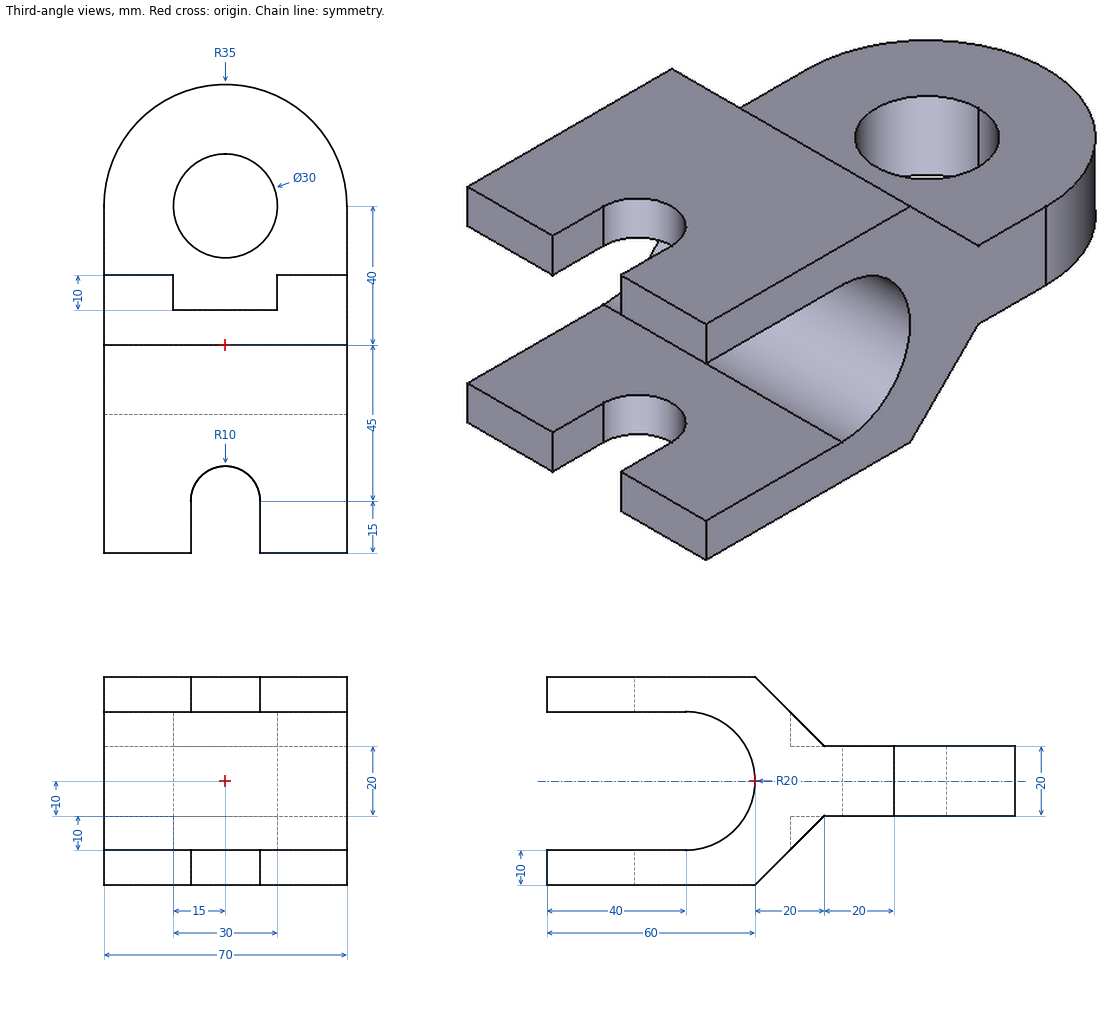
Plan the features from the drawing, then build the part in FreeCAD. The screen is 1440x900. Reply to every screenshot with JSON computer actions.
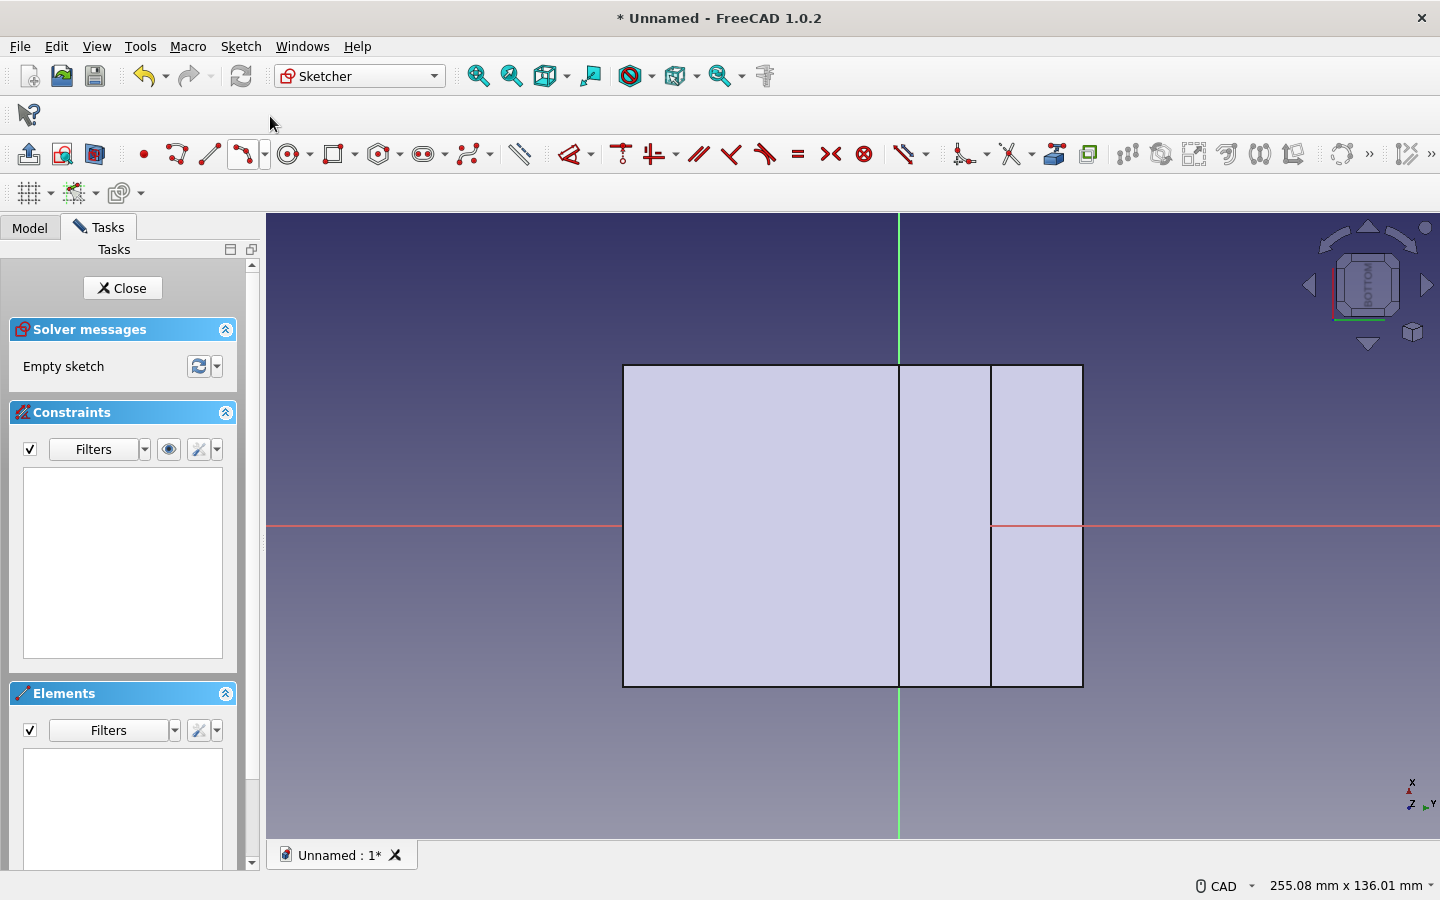
{"action": "key", "text": "g l"}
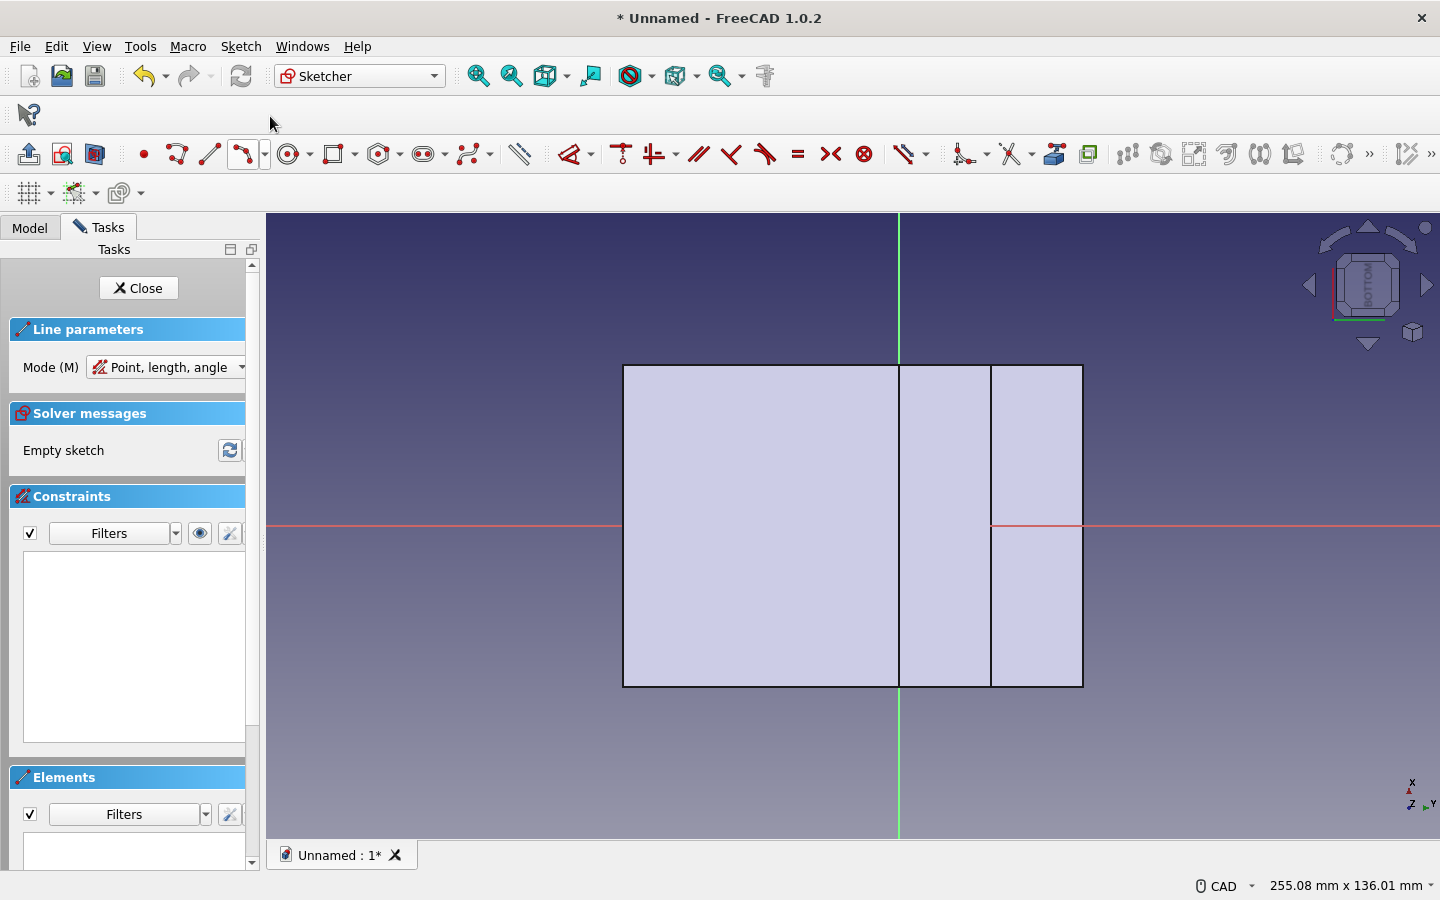
{"action": "left_click", "coordinate": [1083, 365]}
{"action": "left_click", "coordinate": [1083, 687]}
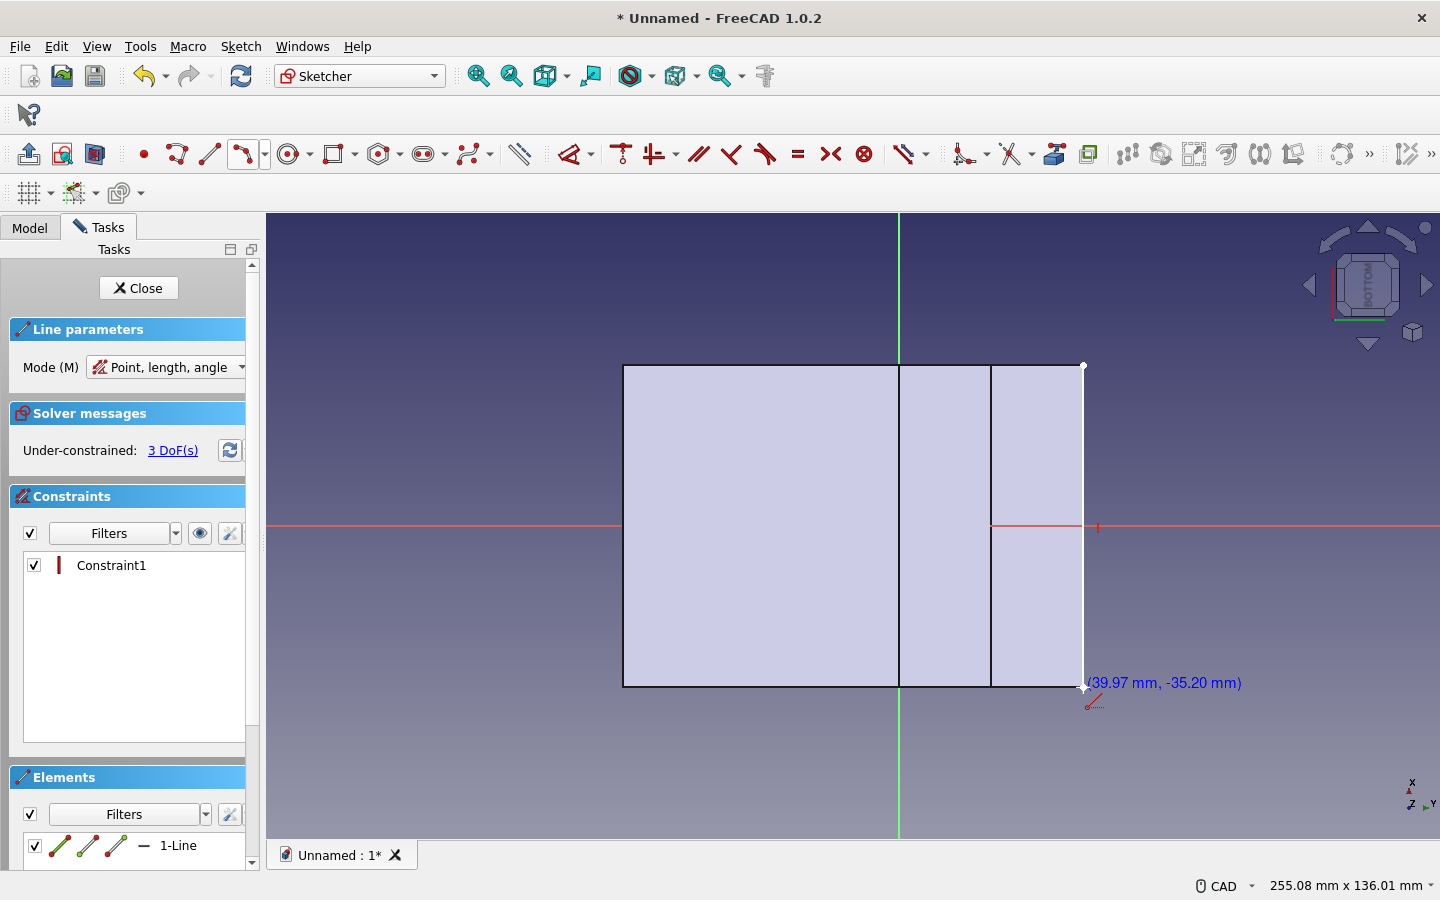
{"action": "left_click", "coordinate": [242, 154]}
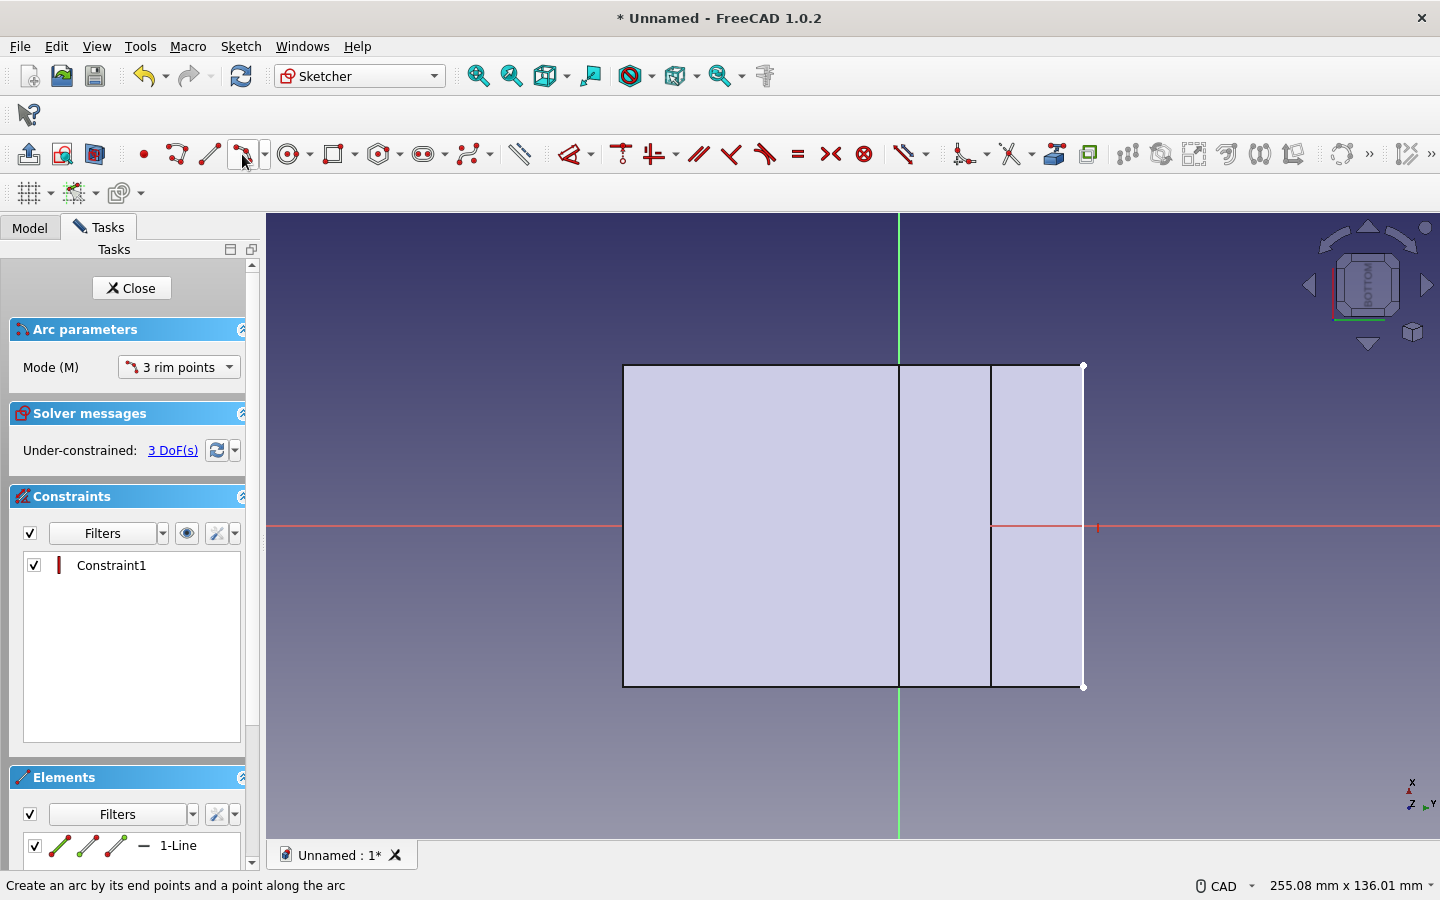
{"action": "left_click", "coordinate": [1083, 688]}
{"action": "left_click", "coordinate": [1083, 366]}
{"action": "left_click", "coordinate": [1236, 576]}
{"action": "key", "text": "Escape"}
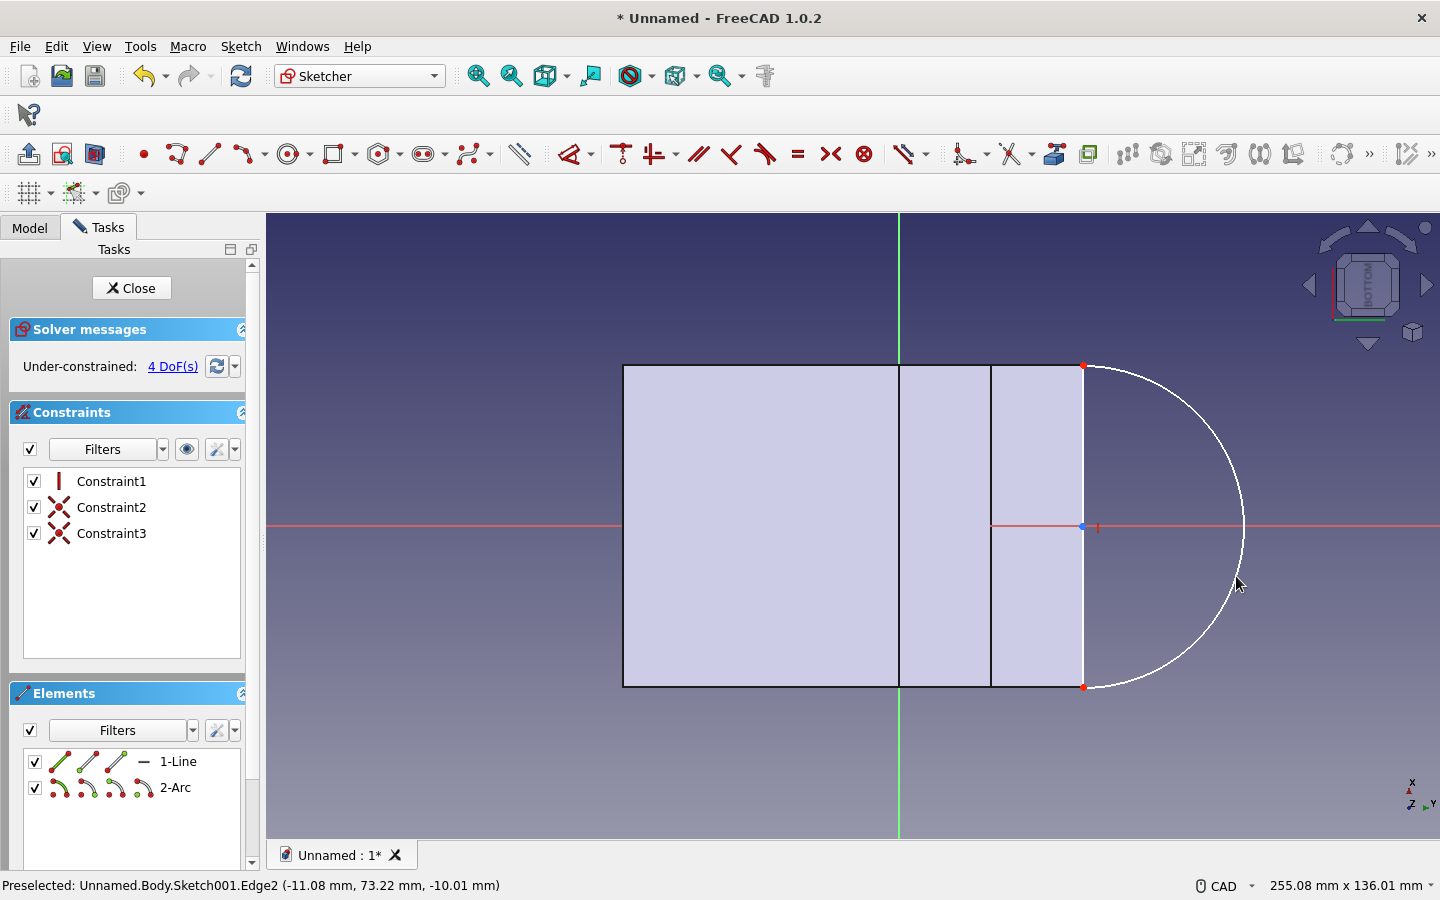
{"action": "left_click", "coordinate": [1083, 527]}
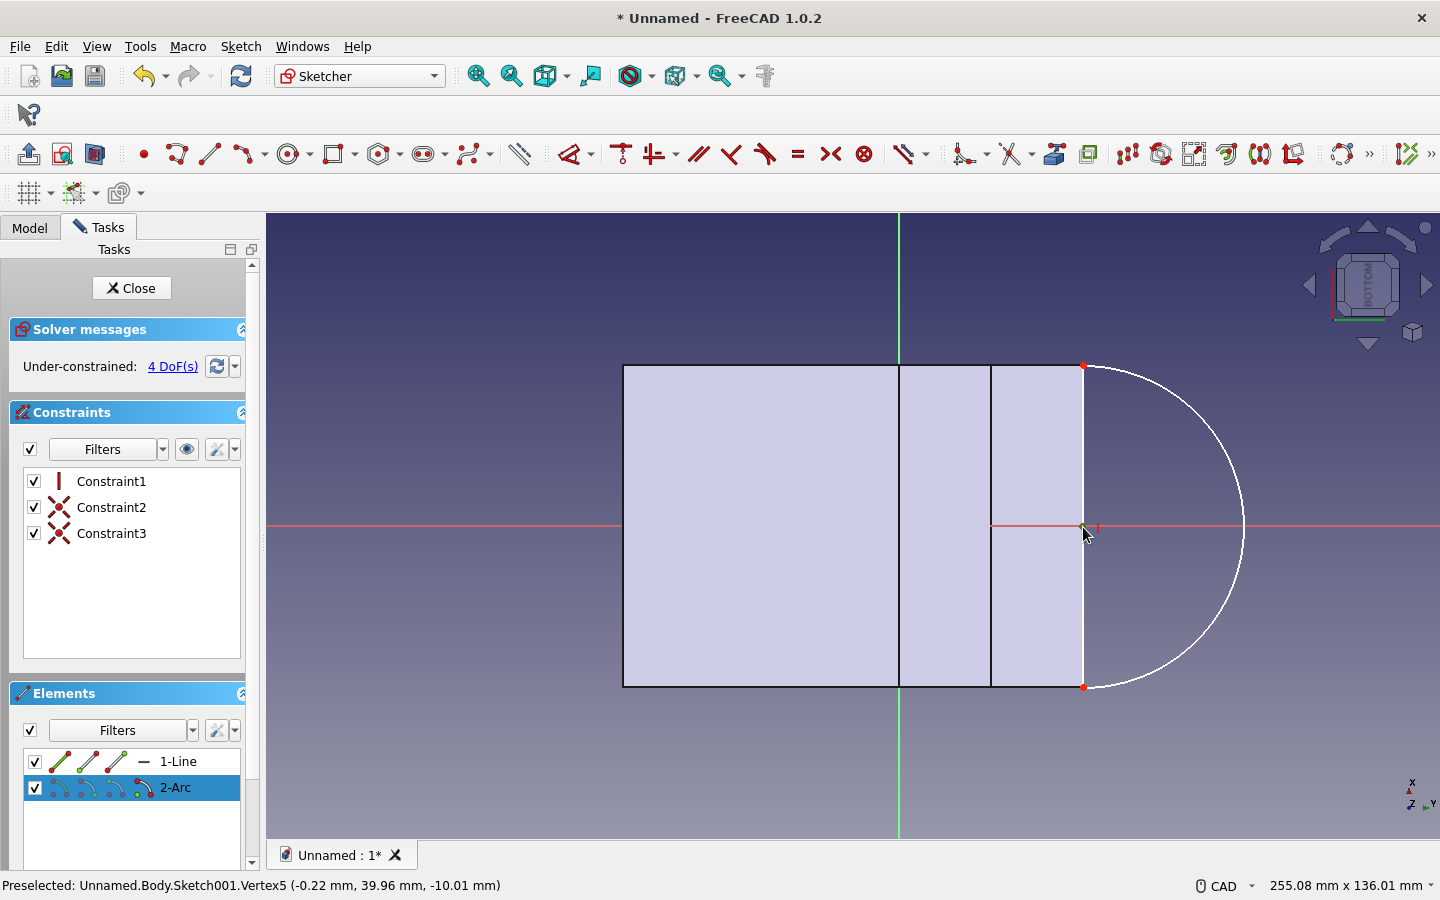
{"action": "left_click", "coordinate": [364, 526]}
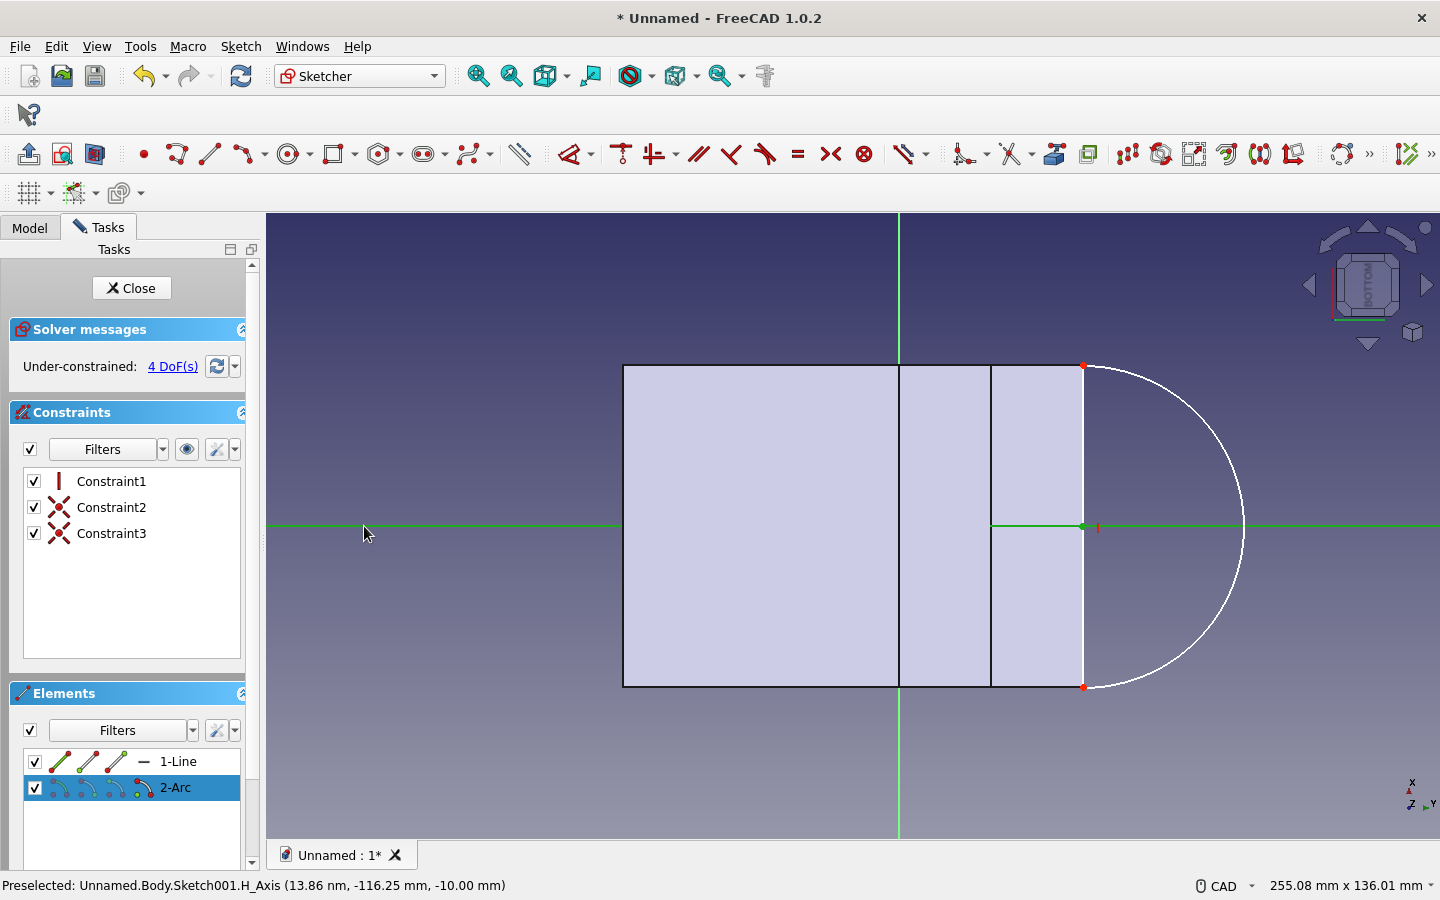
{"action": "key", "text": "c"}